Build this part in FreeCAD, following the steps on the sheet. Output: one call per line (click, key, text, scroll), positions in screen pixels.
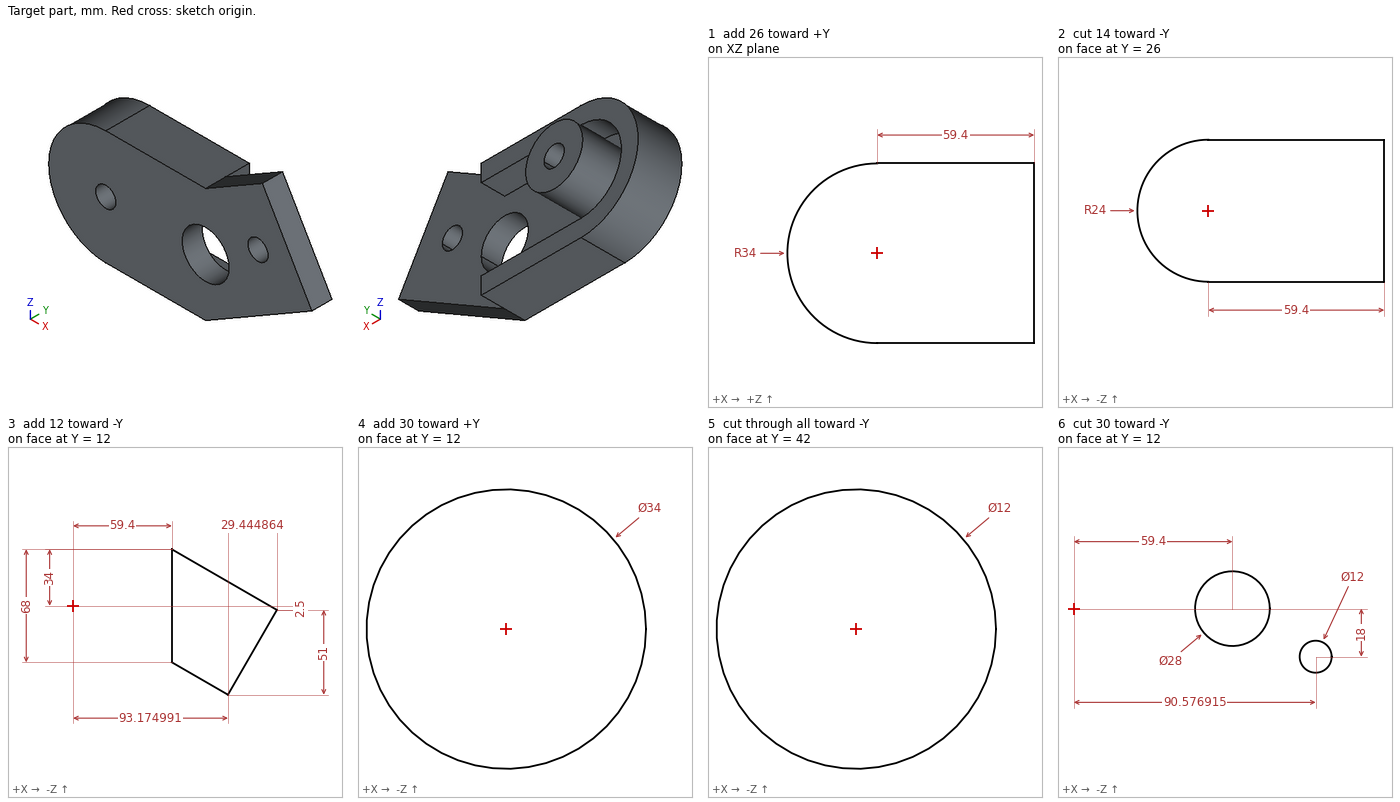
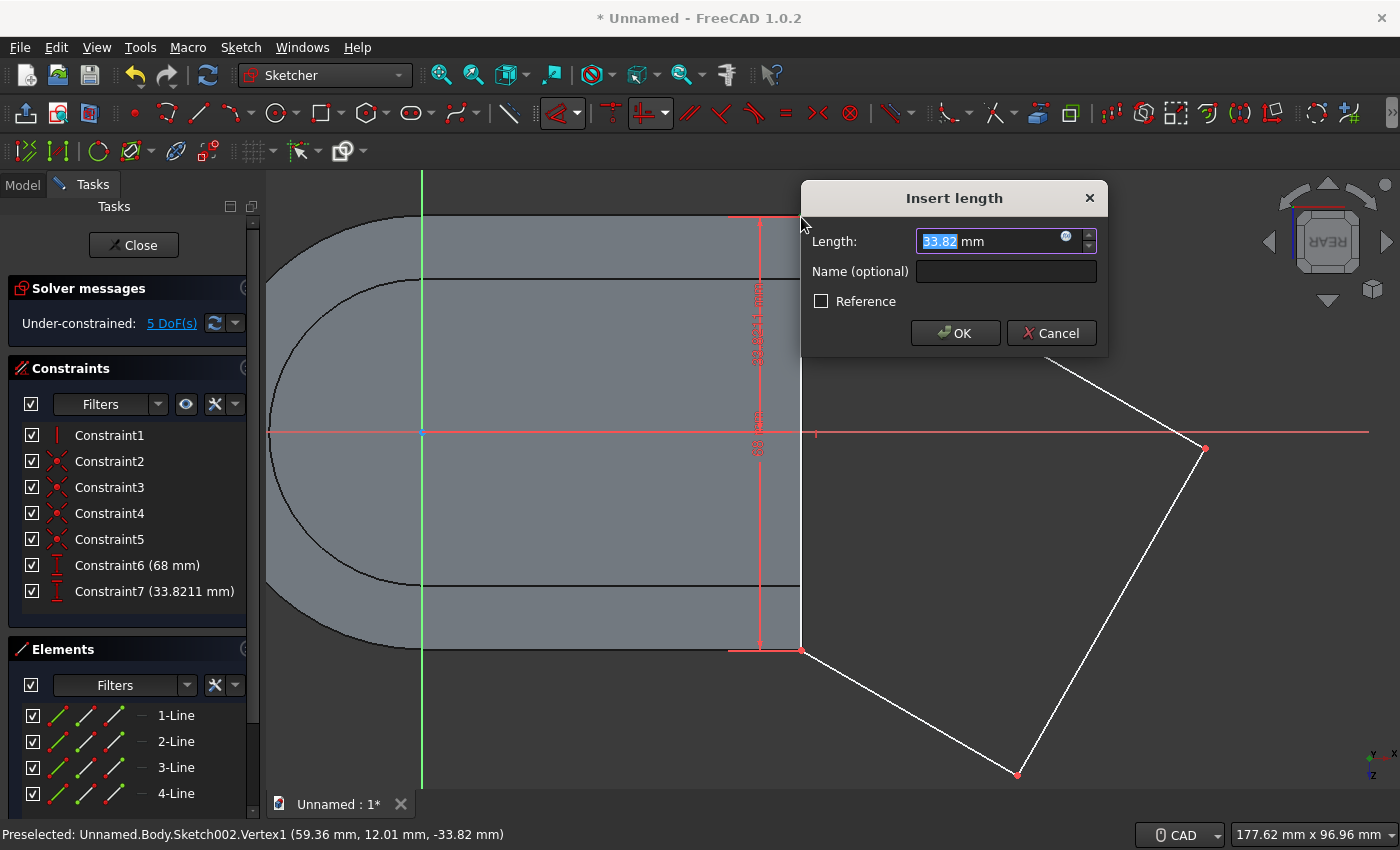
text(34)
key(Return)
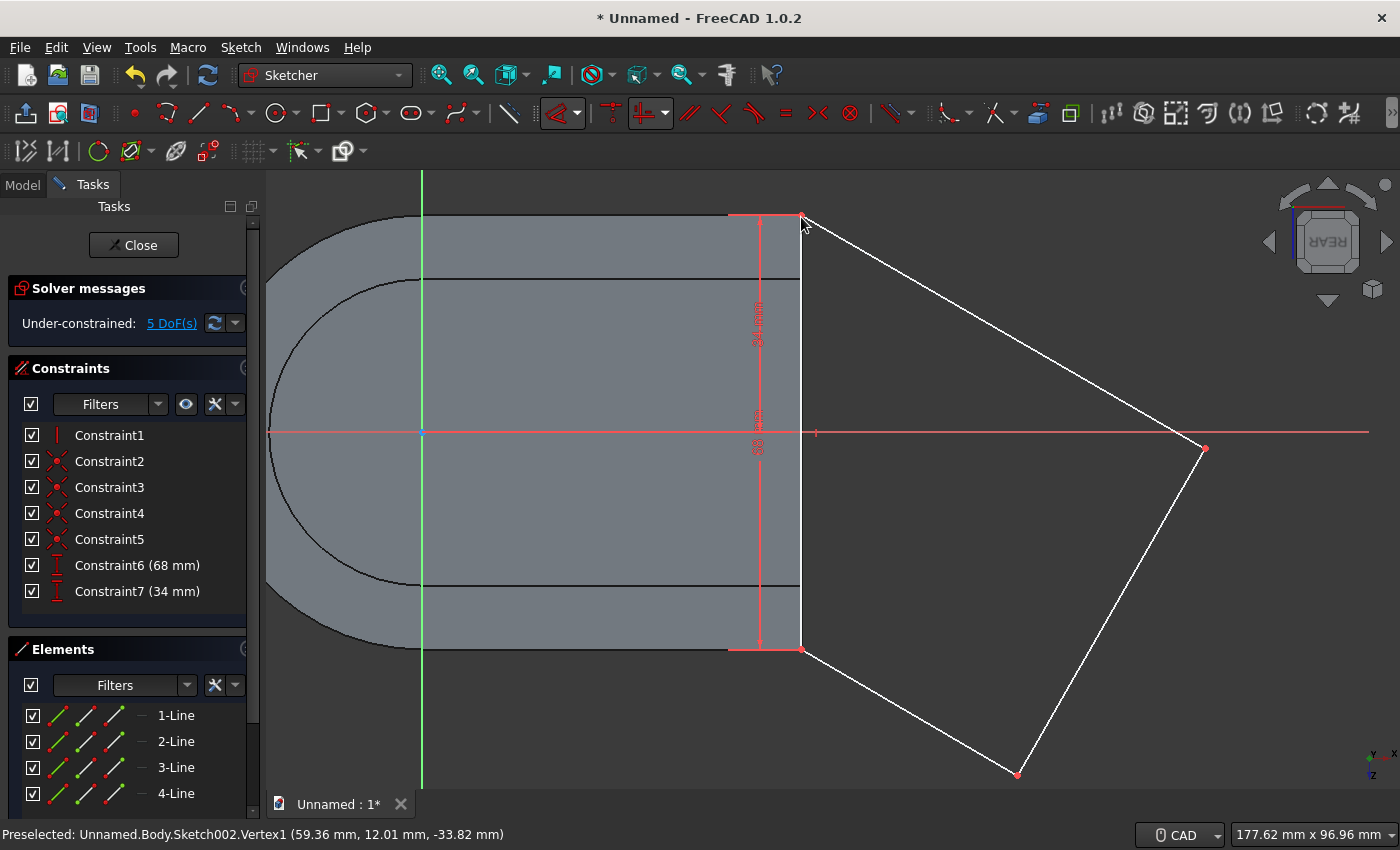
click(1074, 678)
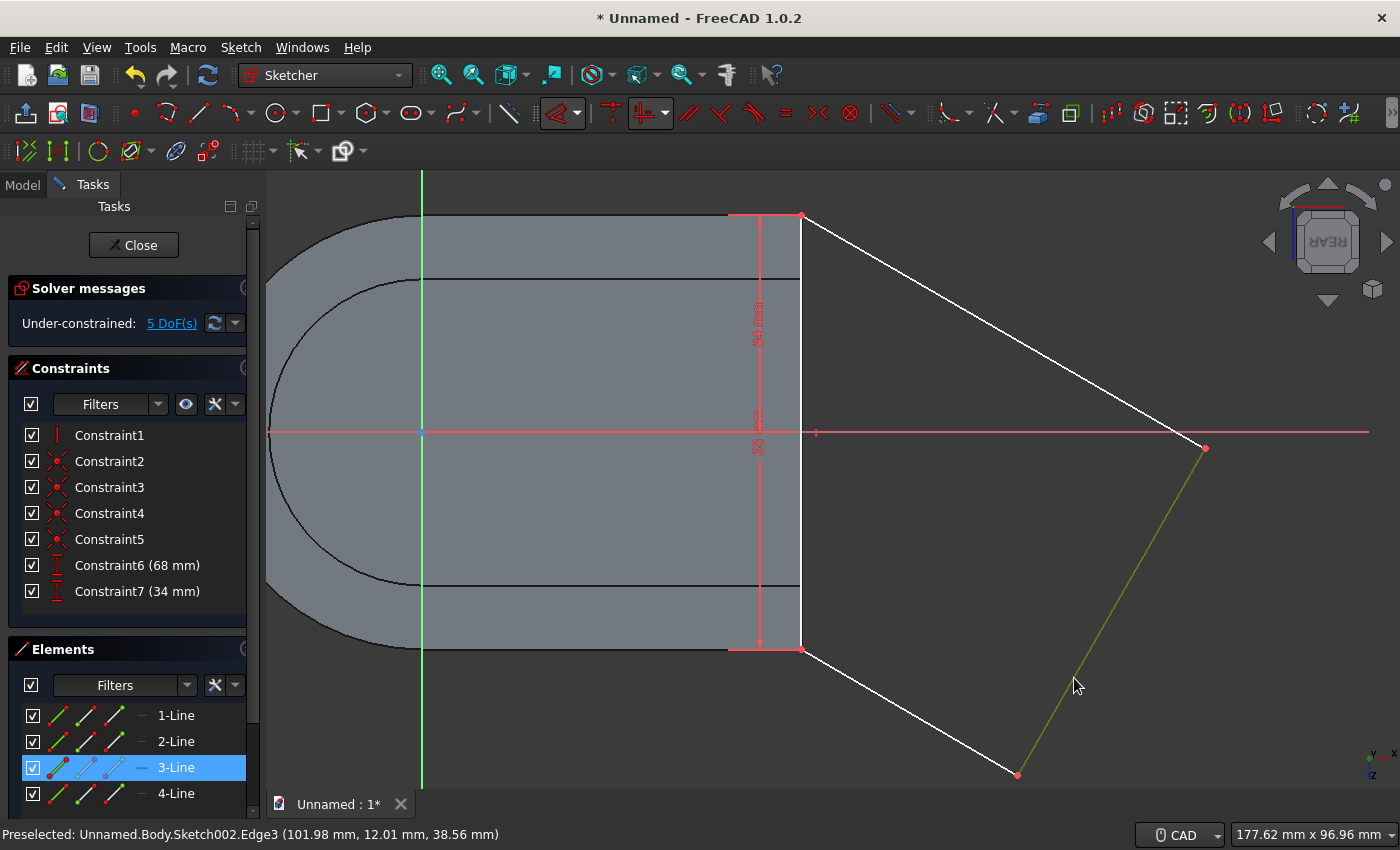
click(580, 114)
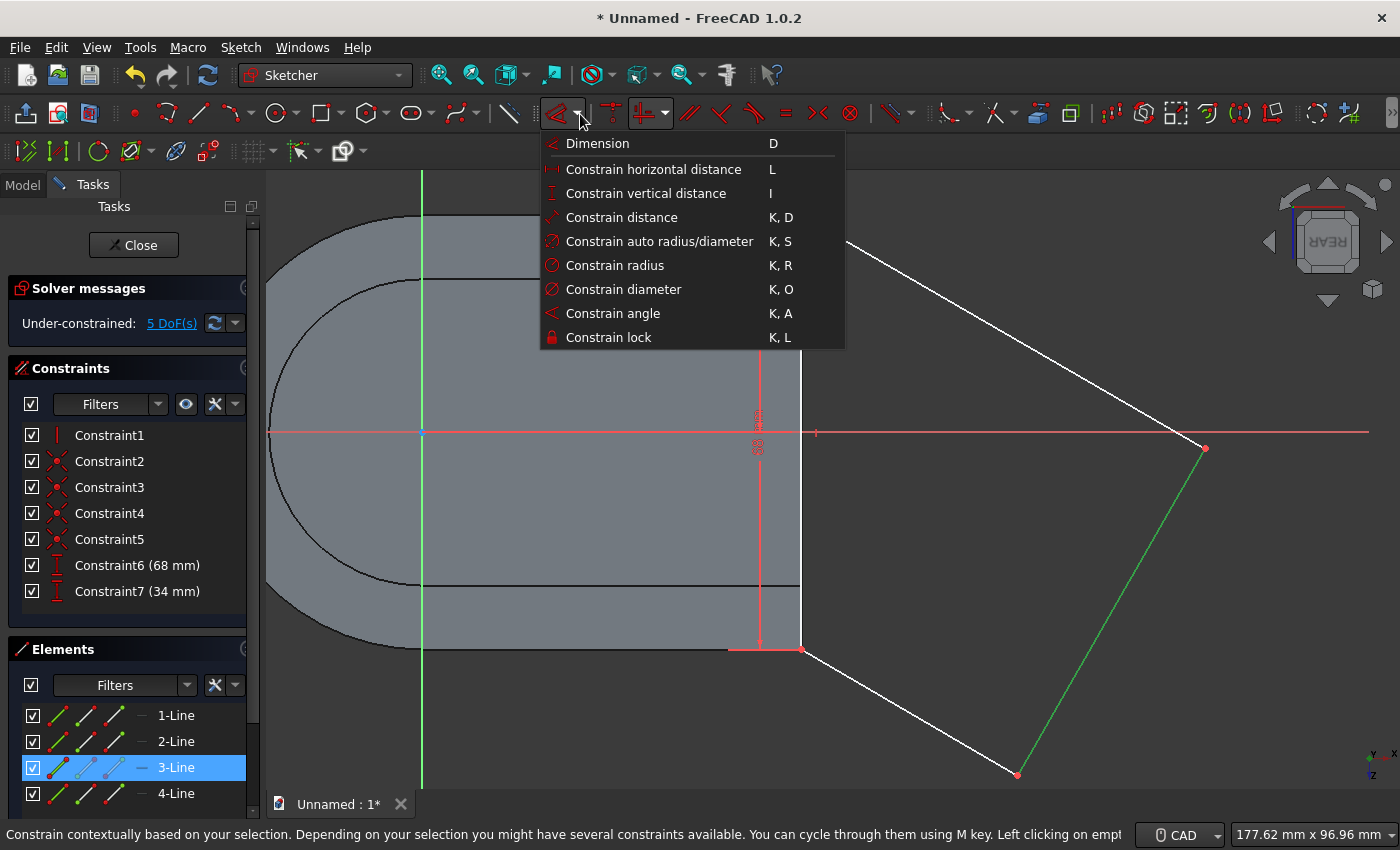
click(693, 193)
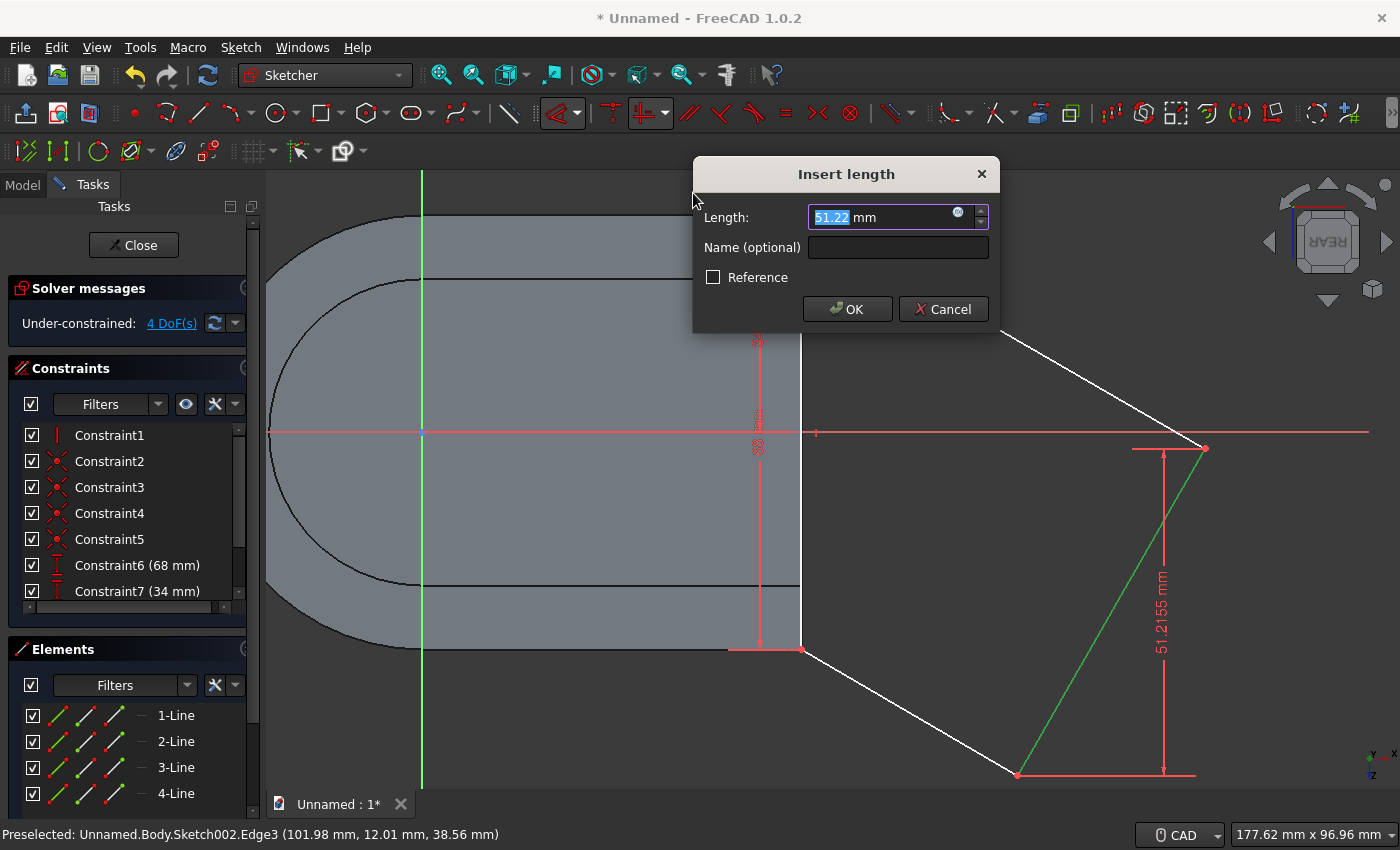
text(51)
key(Return)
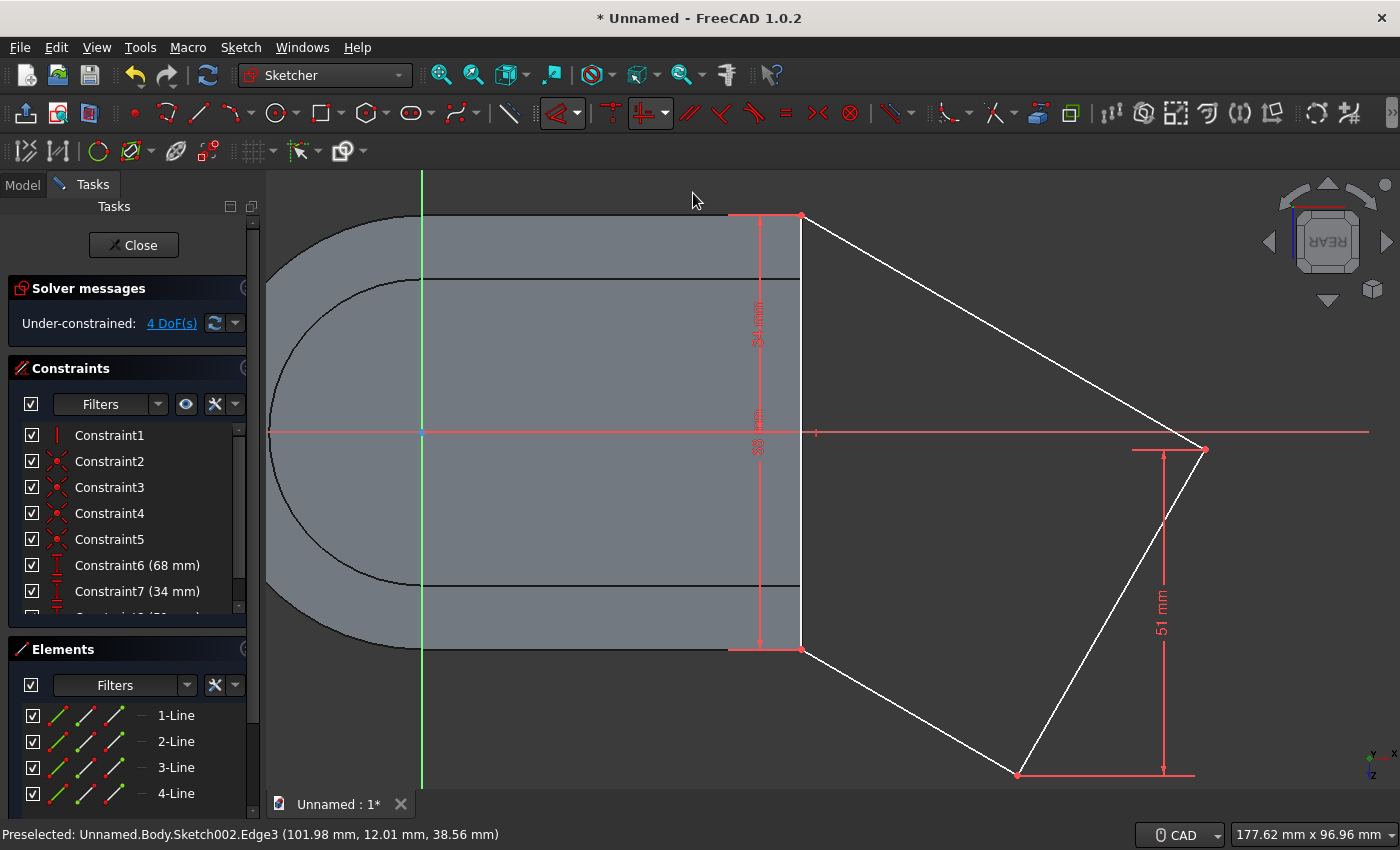
scroll(1205, 450, up, 5)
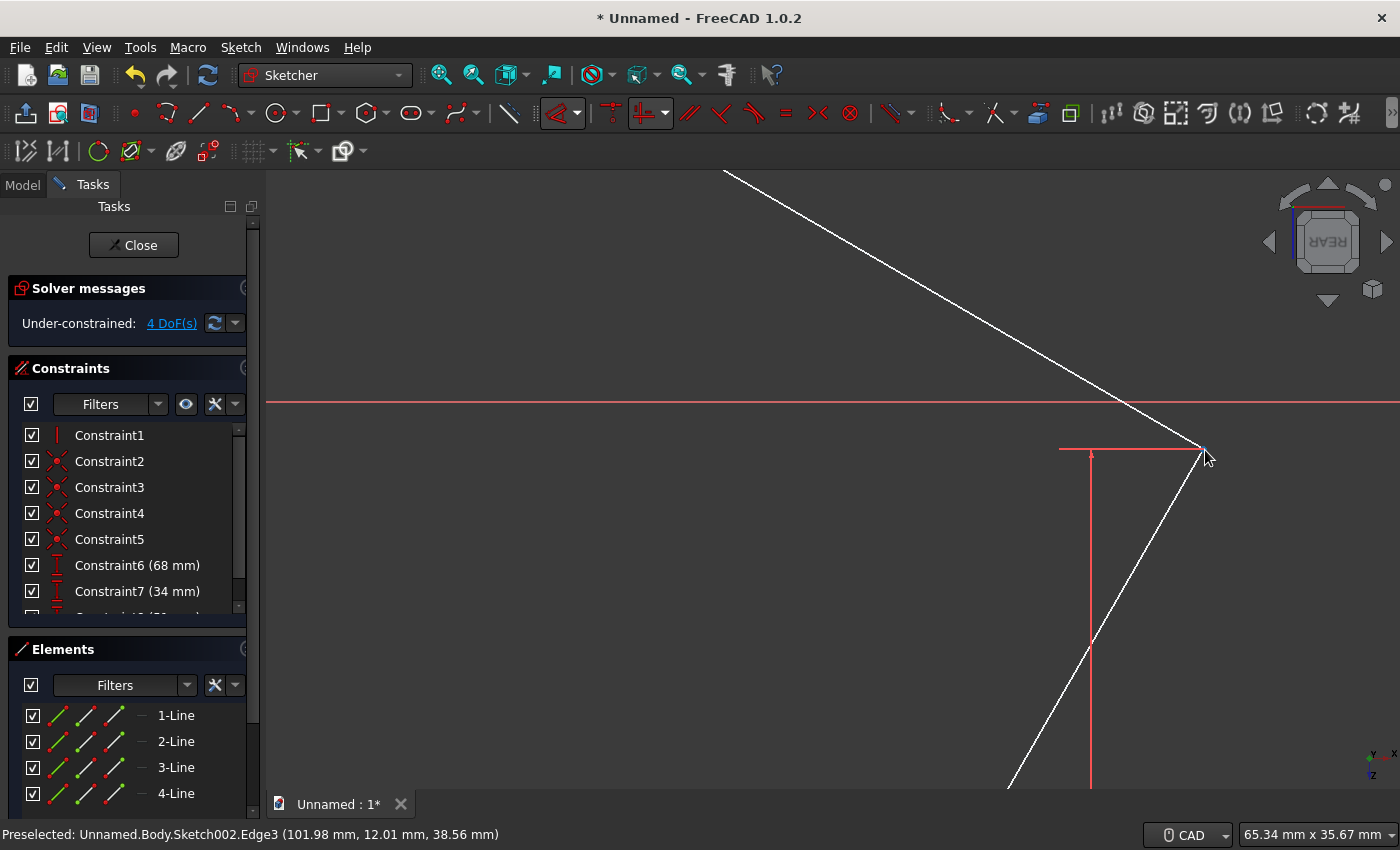
click(1204, 449)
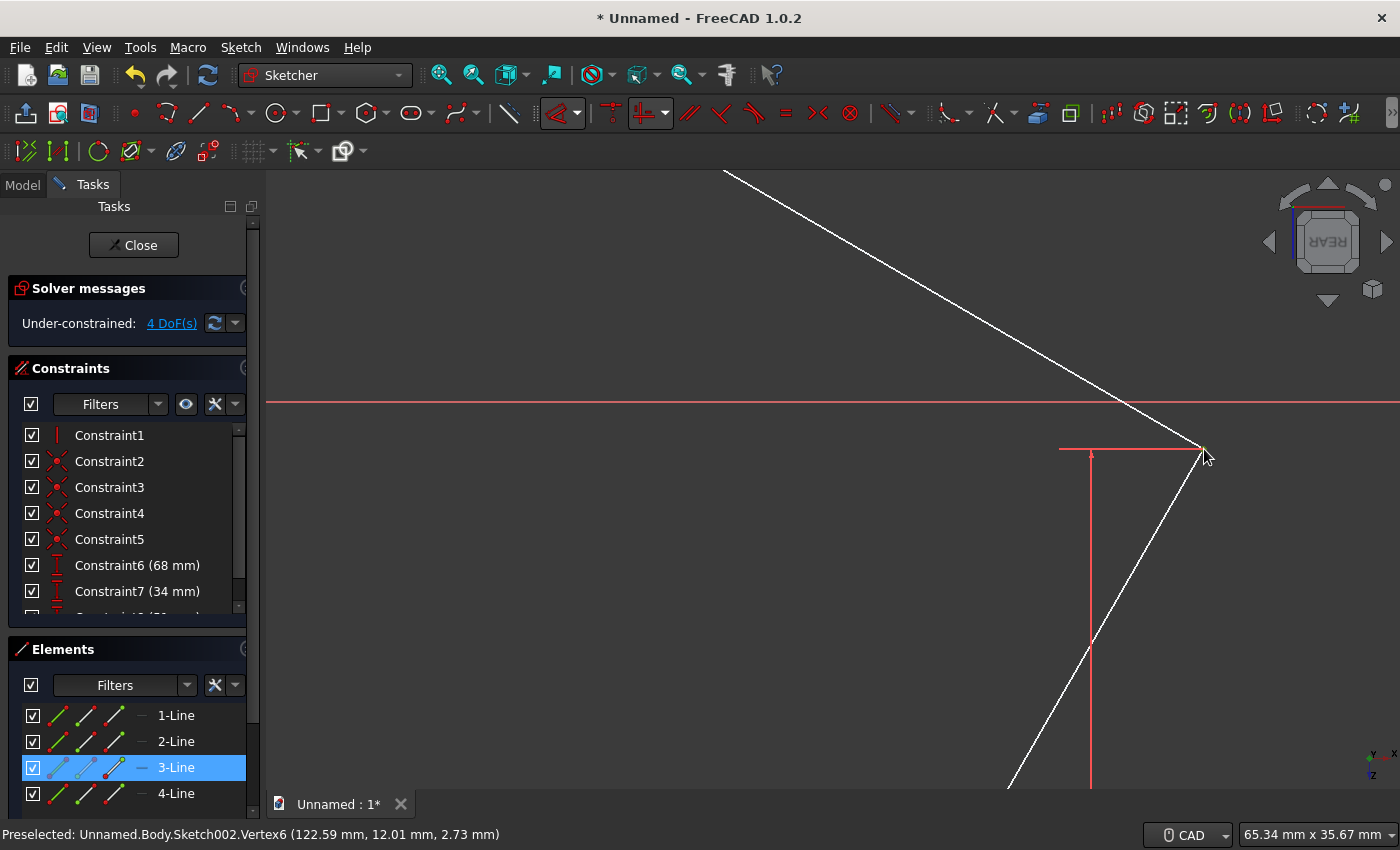
key(i)